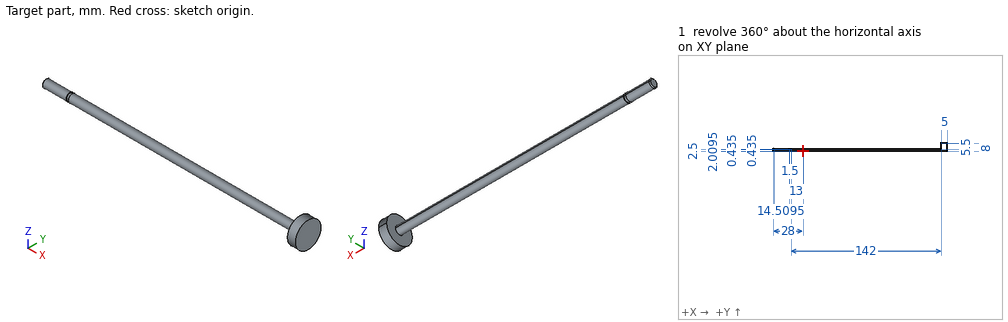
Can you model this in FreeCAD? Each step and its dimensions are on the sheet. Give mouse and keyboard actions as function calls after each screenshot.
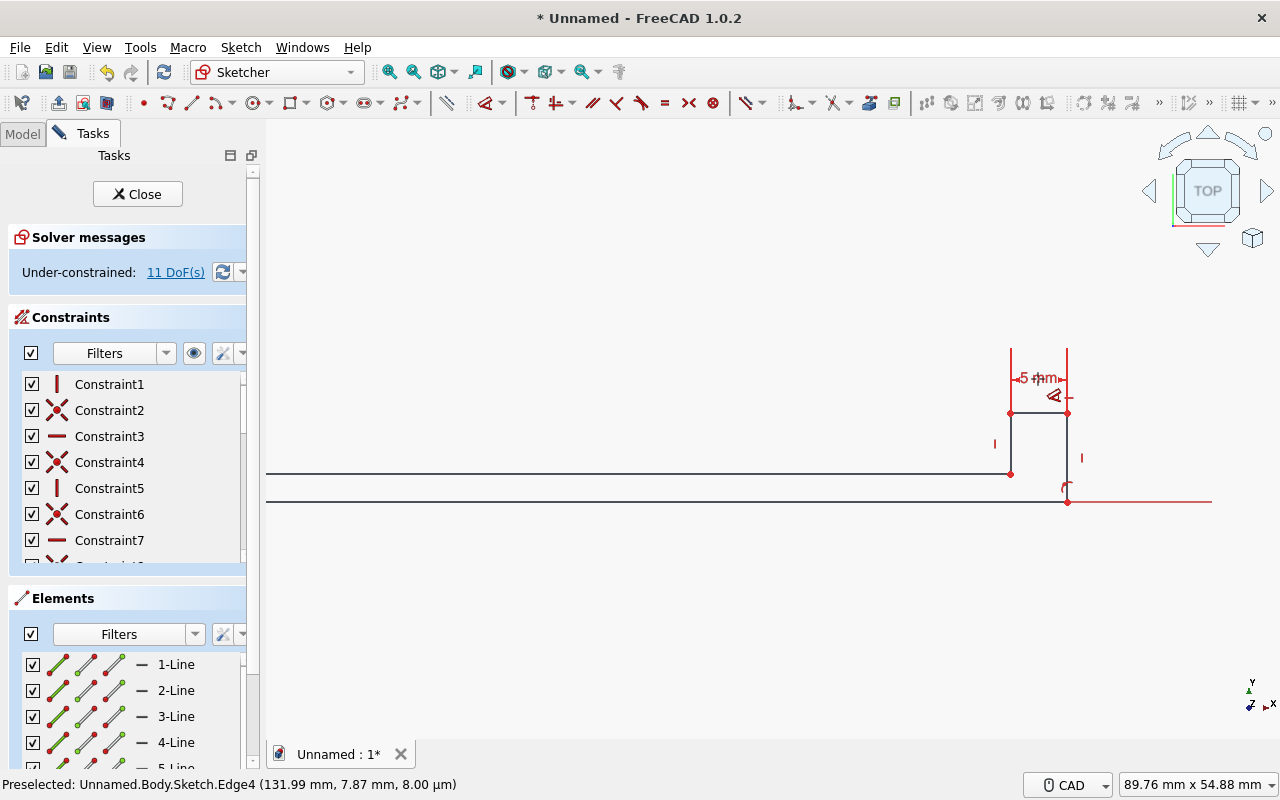
click(1067, 440)
click(1101, 458)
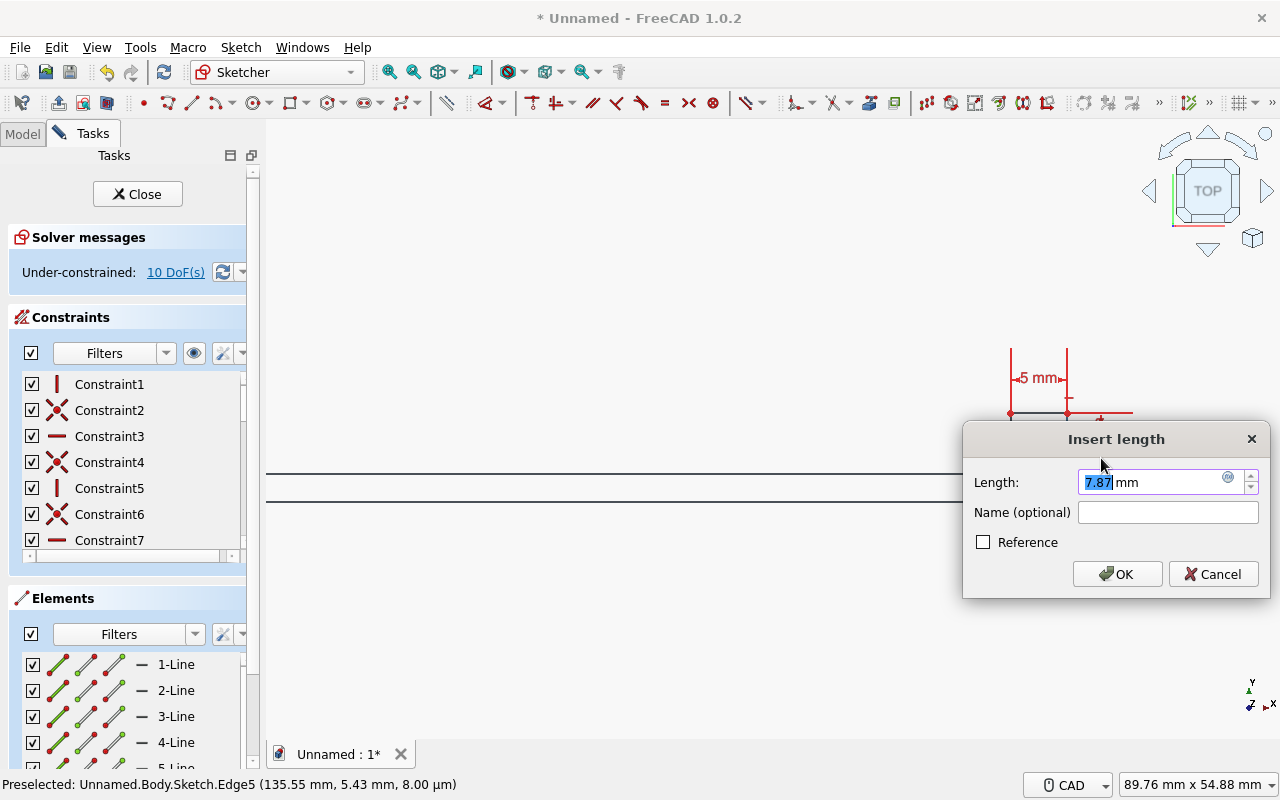
text(8)
key(Return)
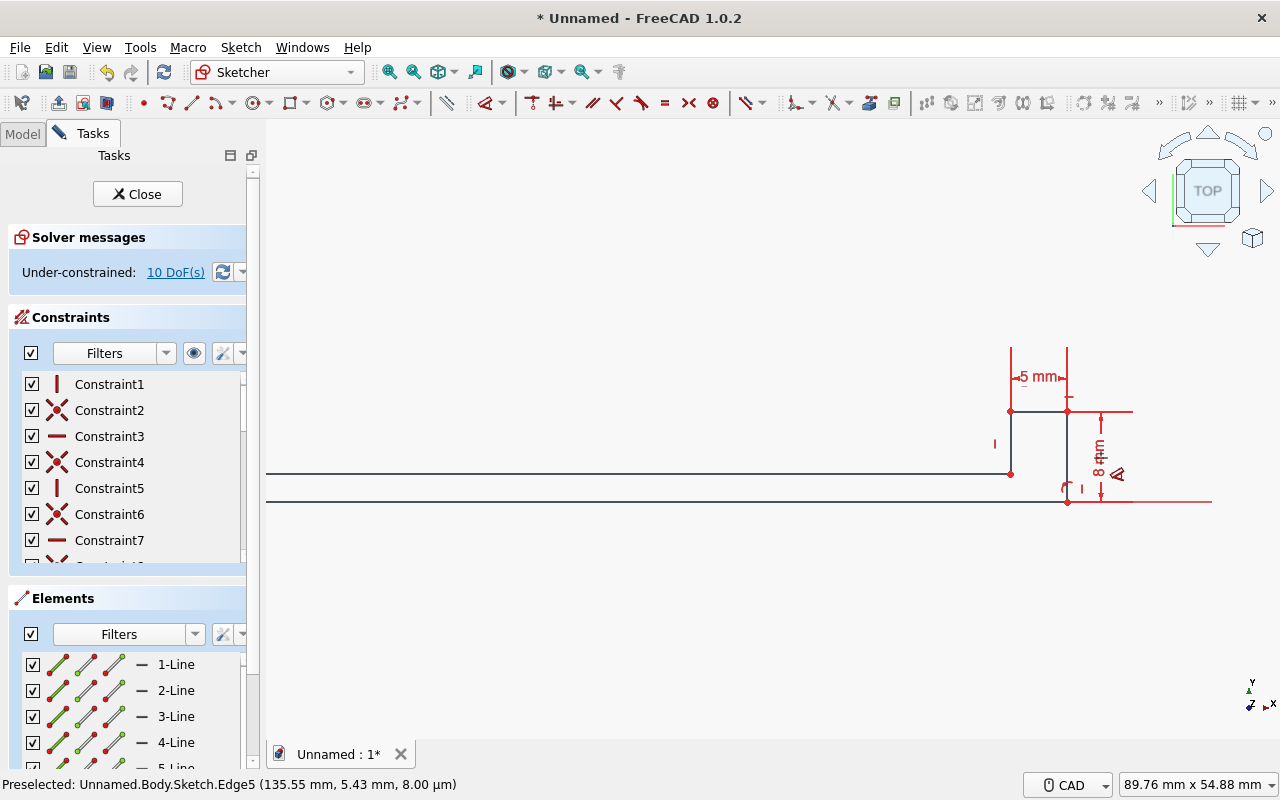
click(529, 474)
click(652, 440)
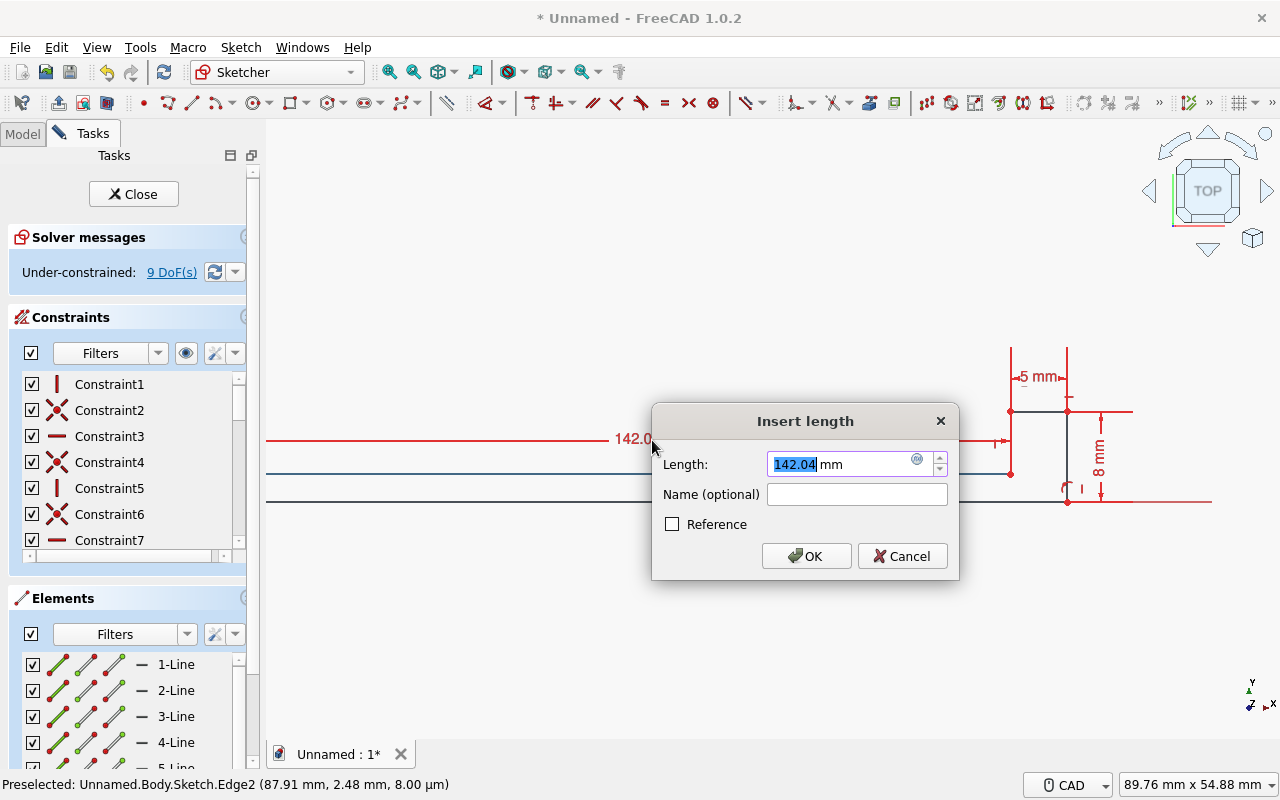
text(142)
key(Return)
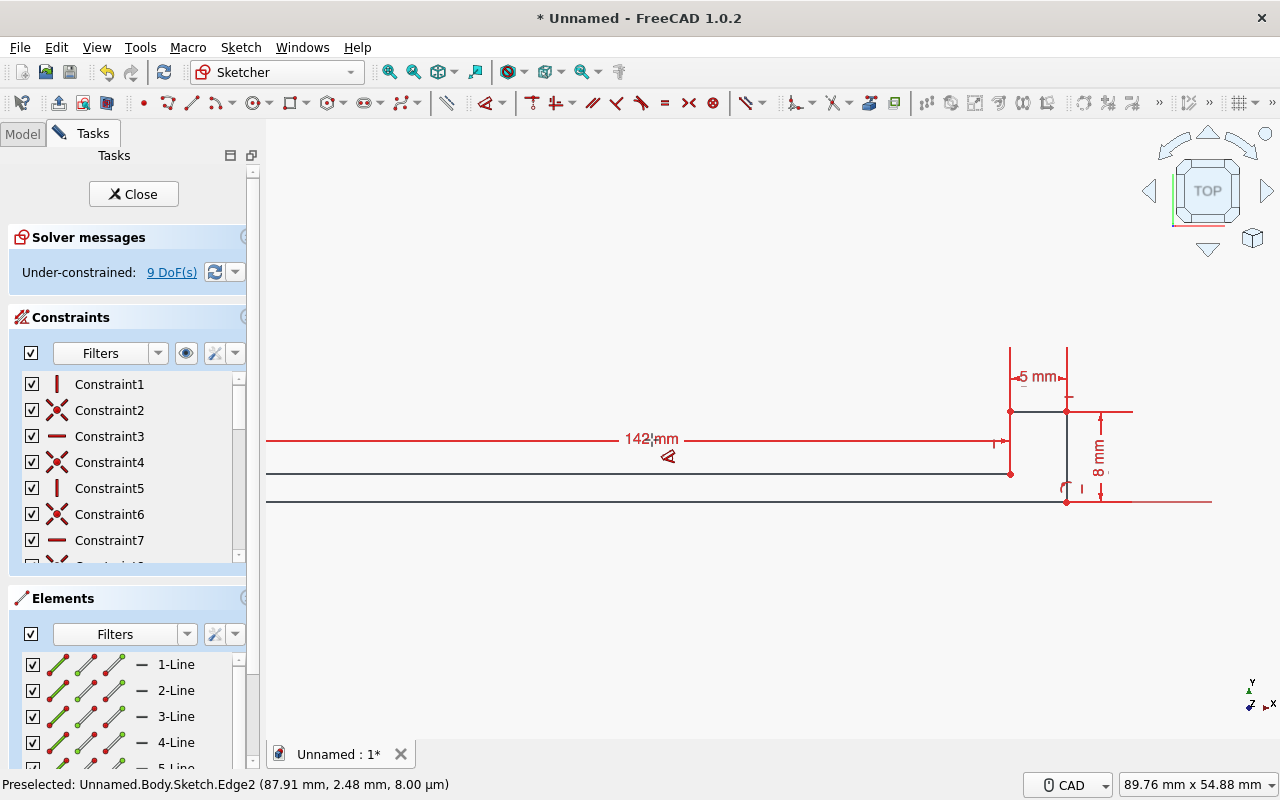
click(1010, 456)
click(1044, 429)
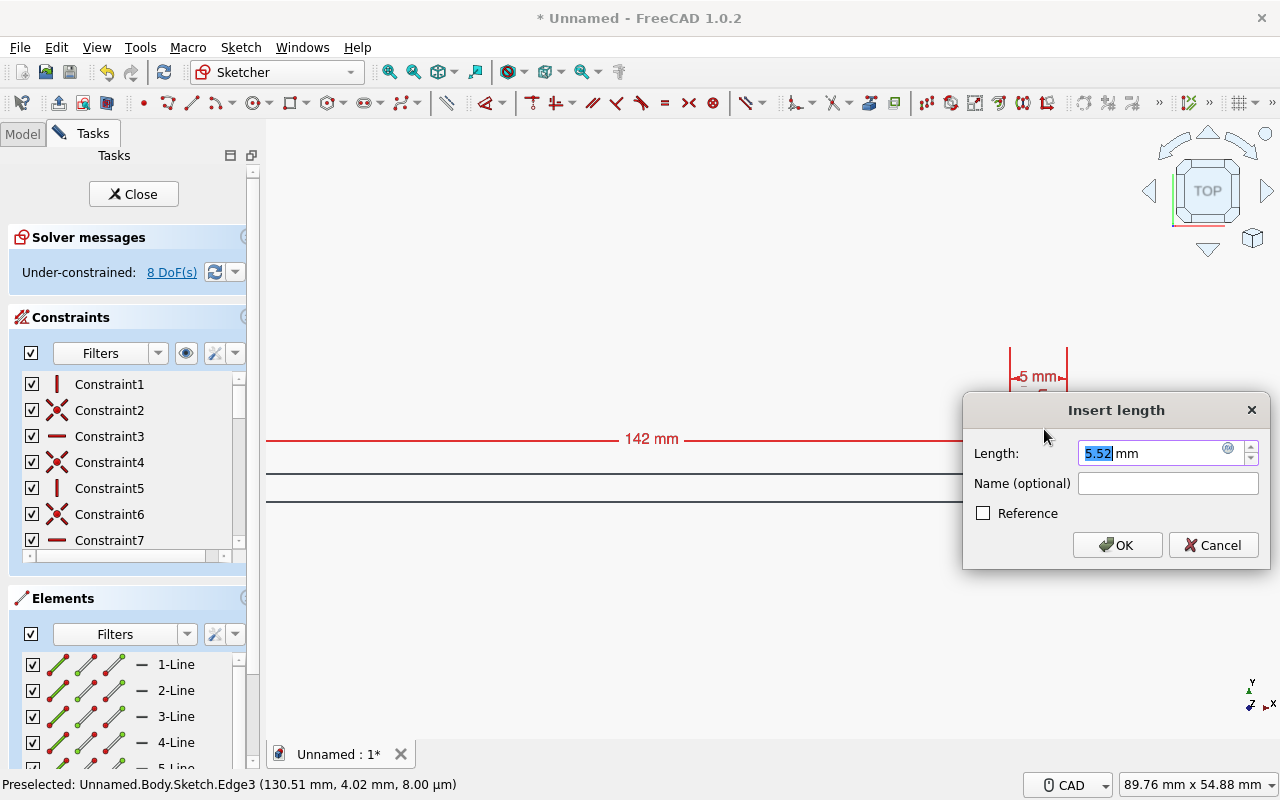
text(5.5)
key(Return)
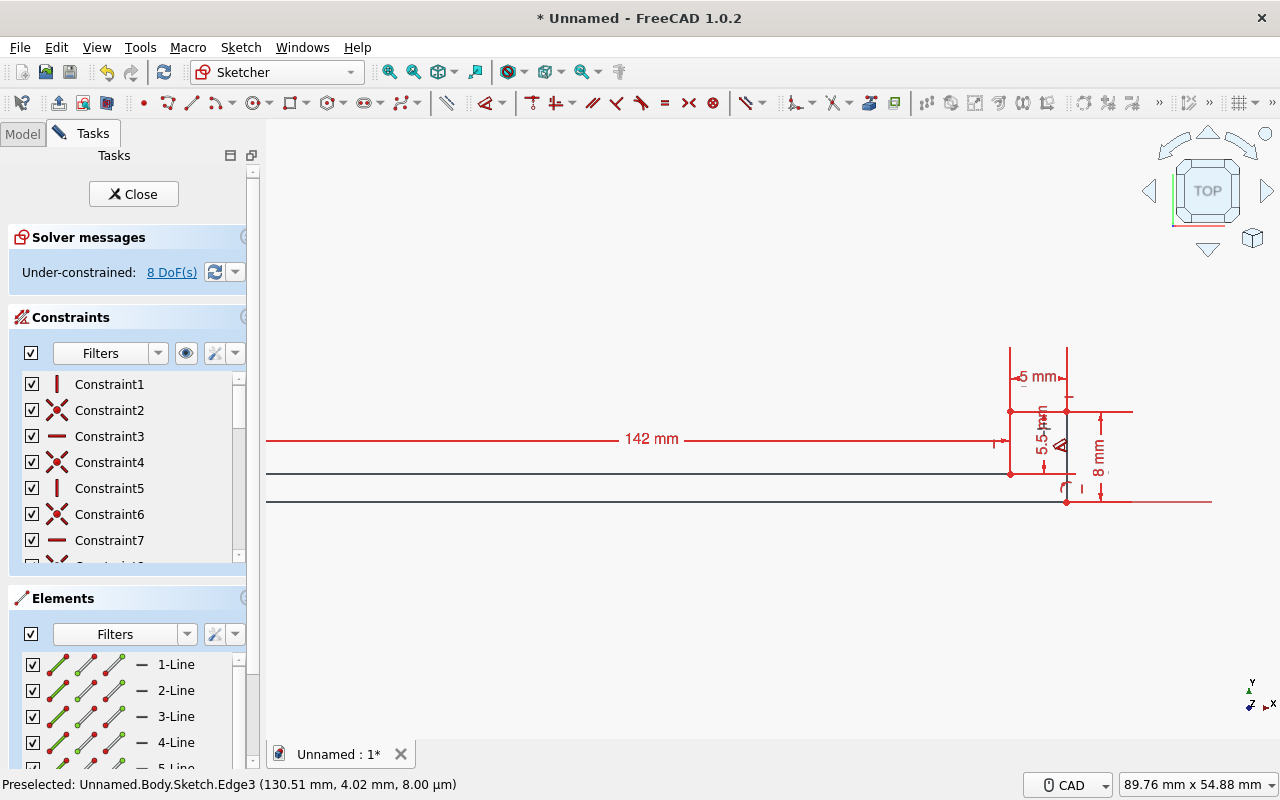
scroll(946, 417, down, 6)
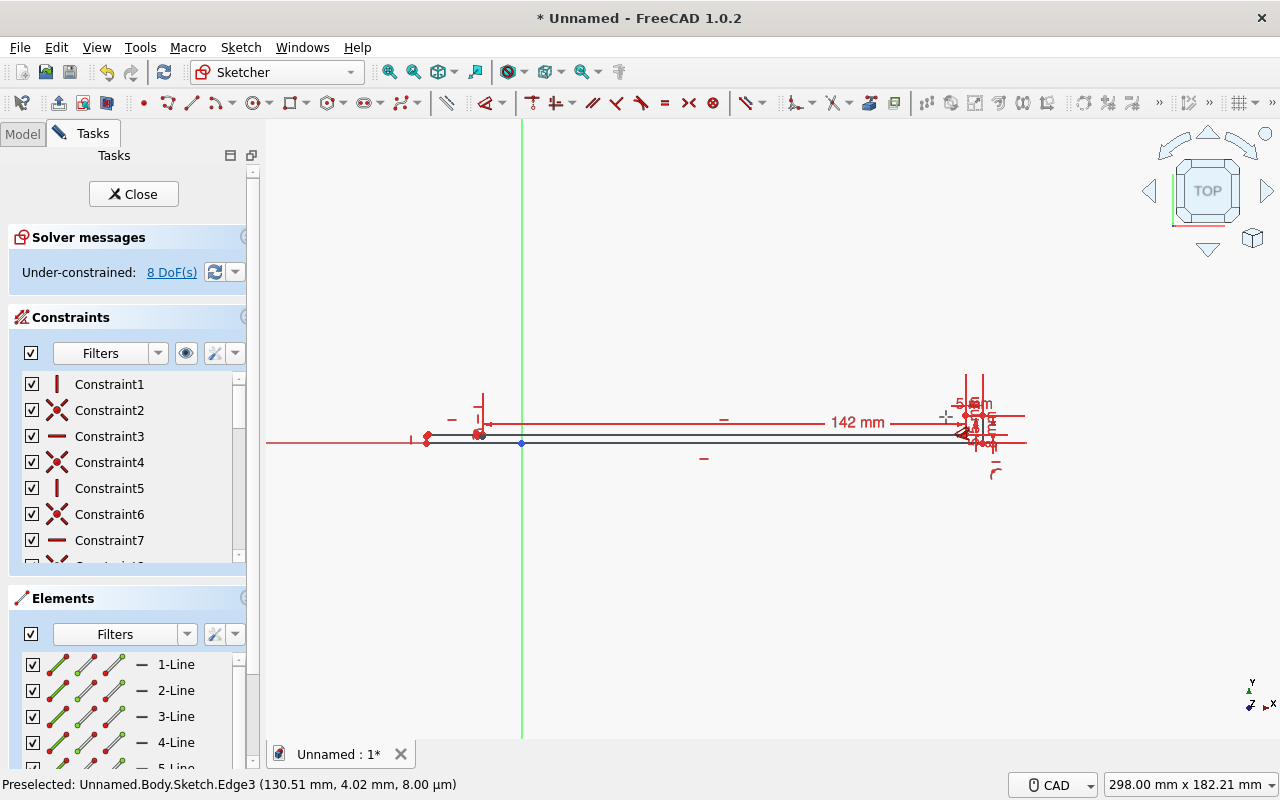
scroll(480, 436, up, 11)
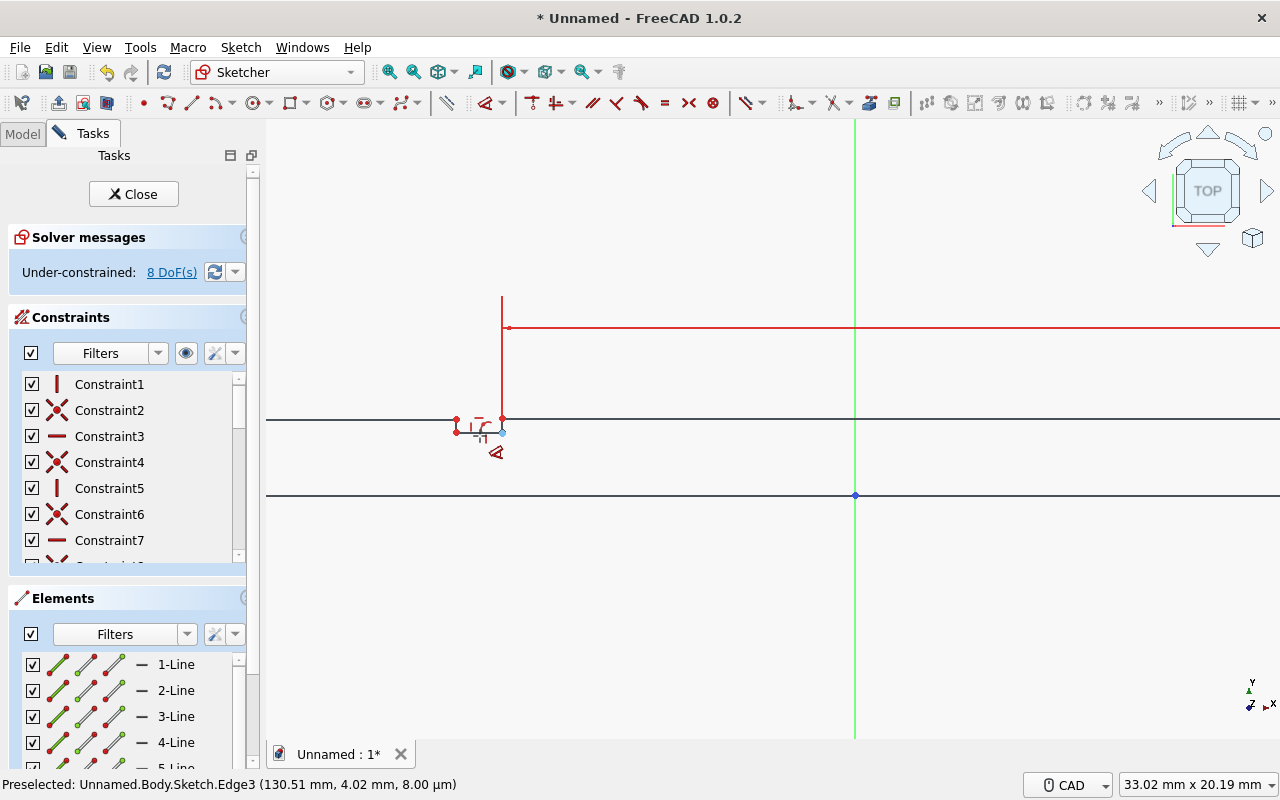
click(479, 433)
click(479, 467)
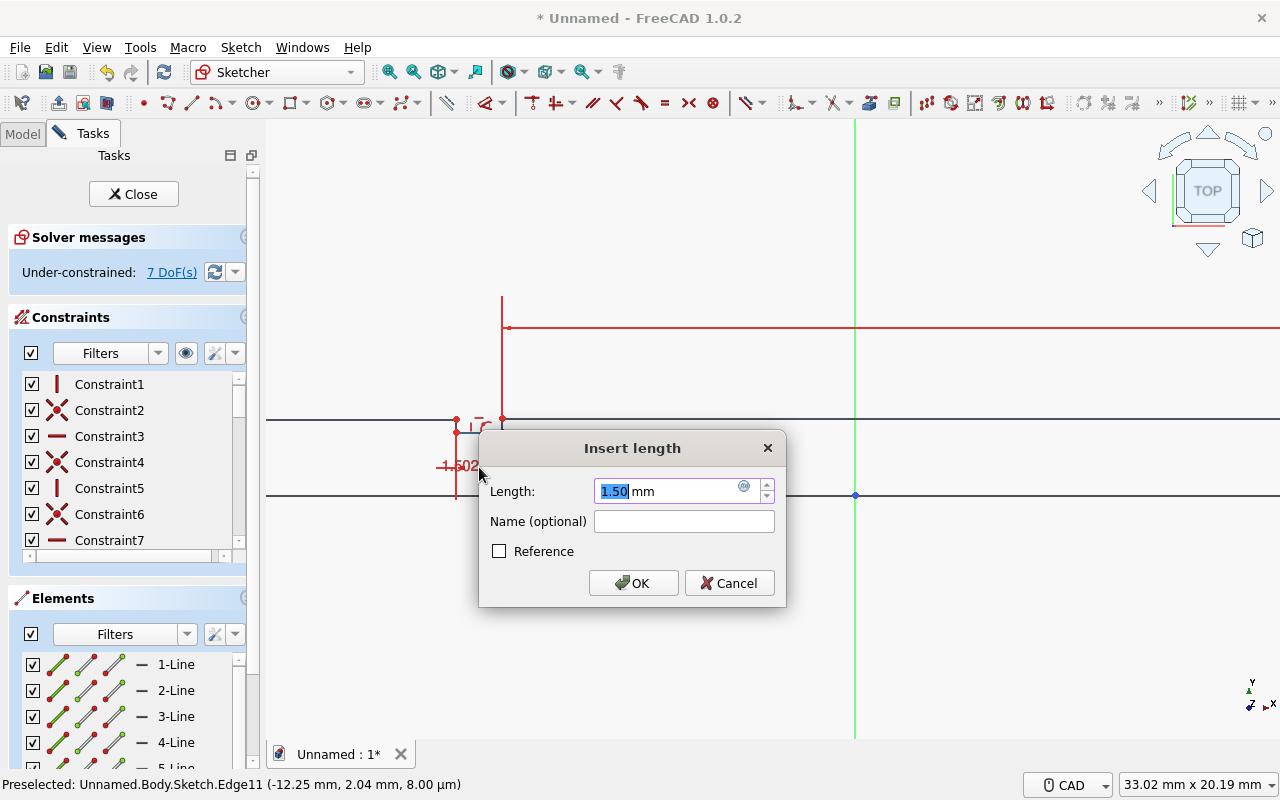
text(1.5)
key(Return)